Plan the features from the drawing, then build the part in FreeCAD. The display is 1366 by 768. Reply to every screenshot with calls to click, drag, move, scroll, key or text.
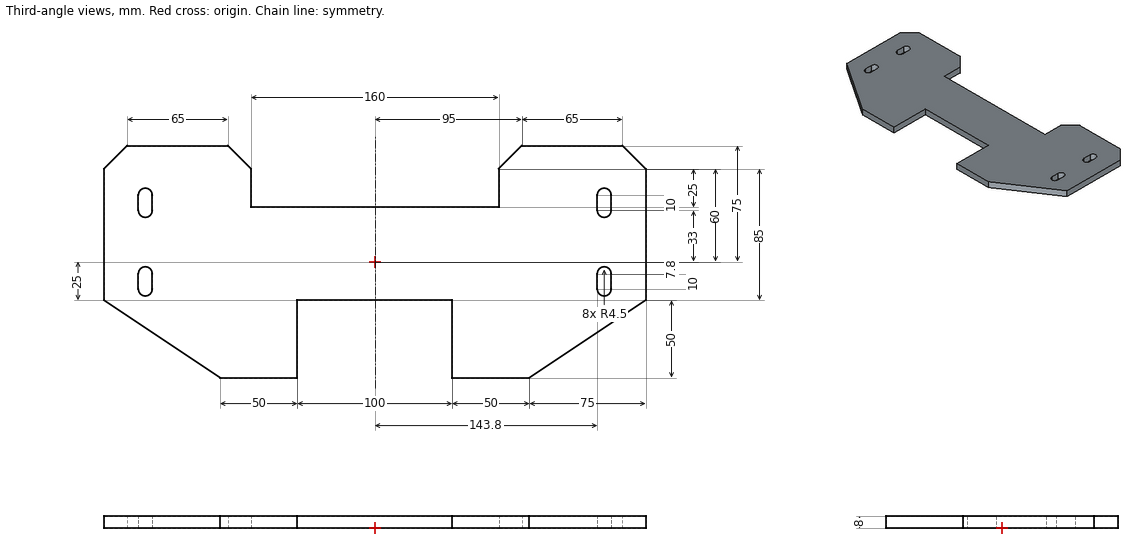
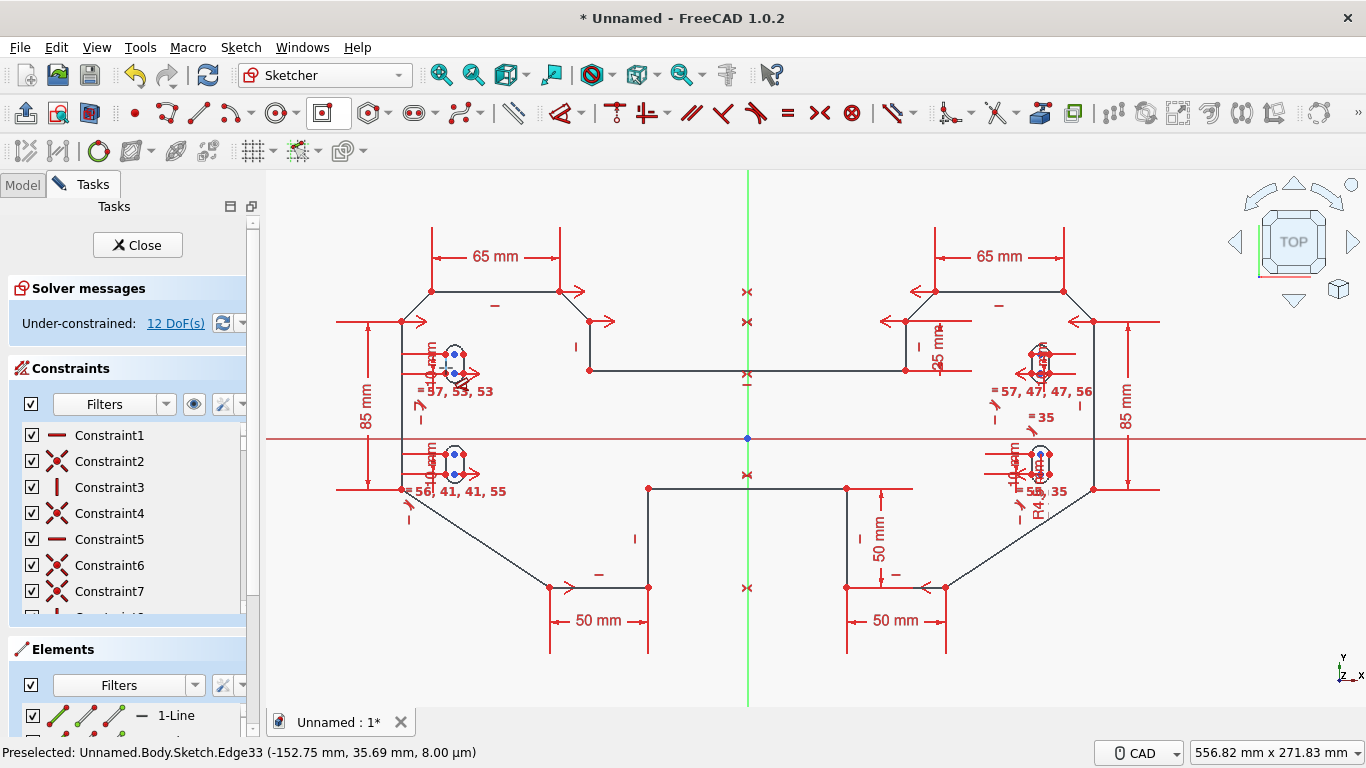
click(708, 489)
click(702, 523)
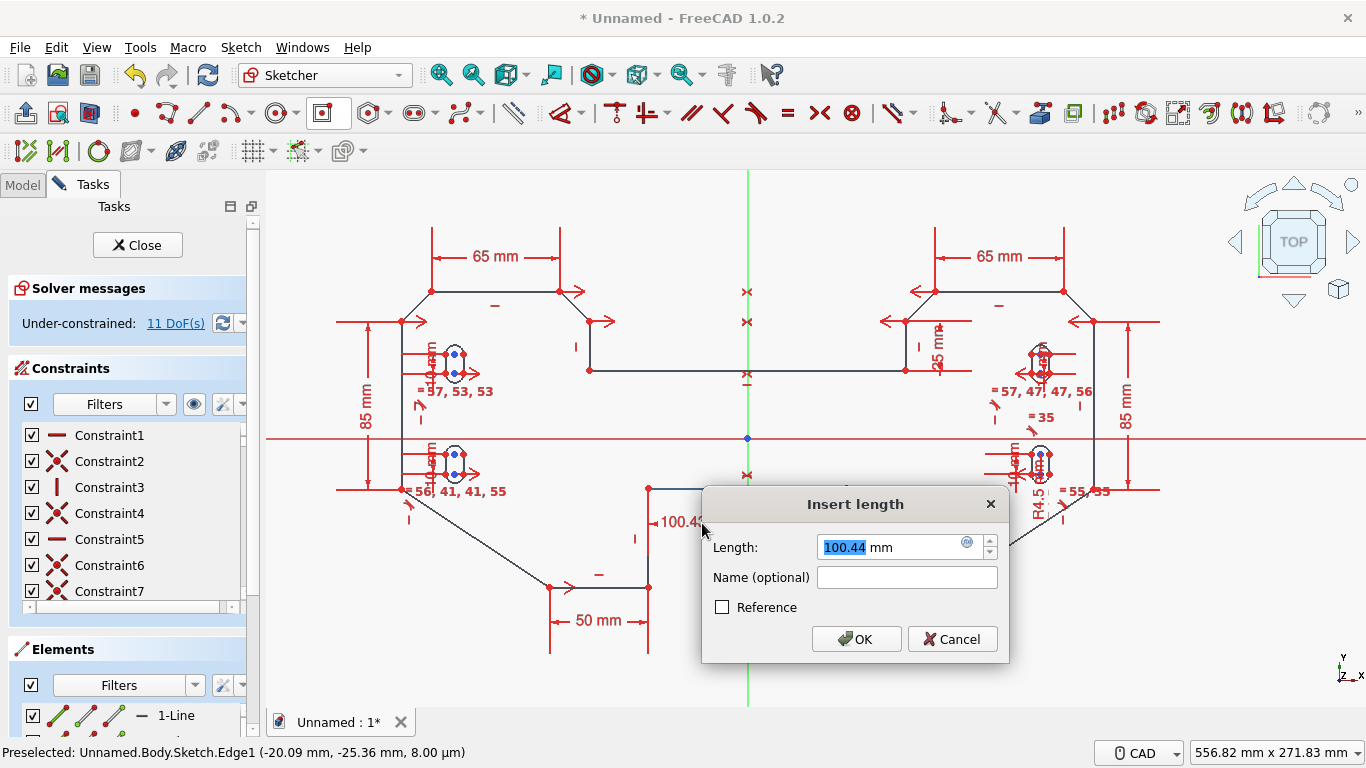
text(100)
key(Return)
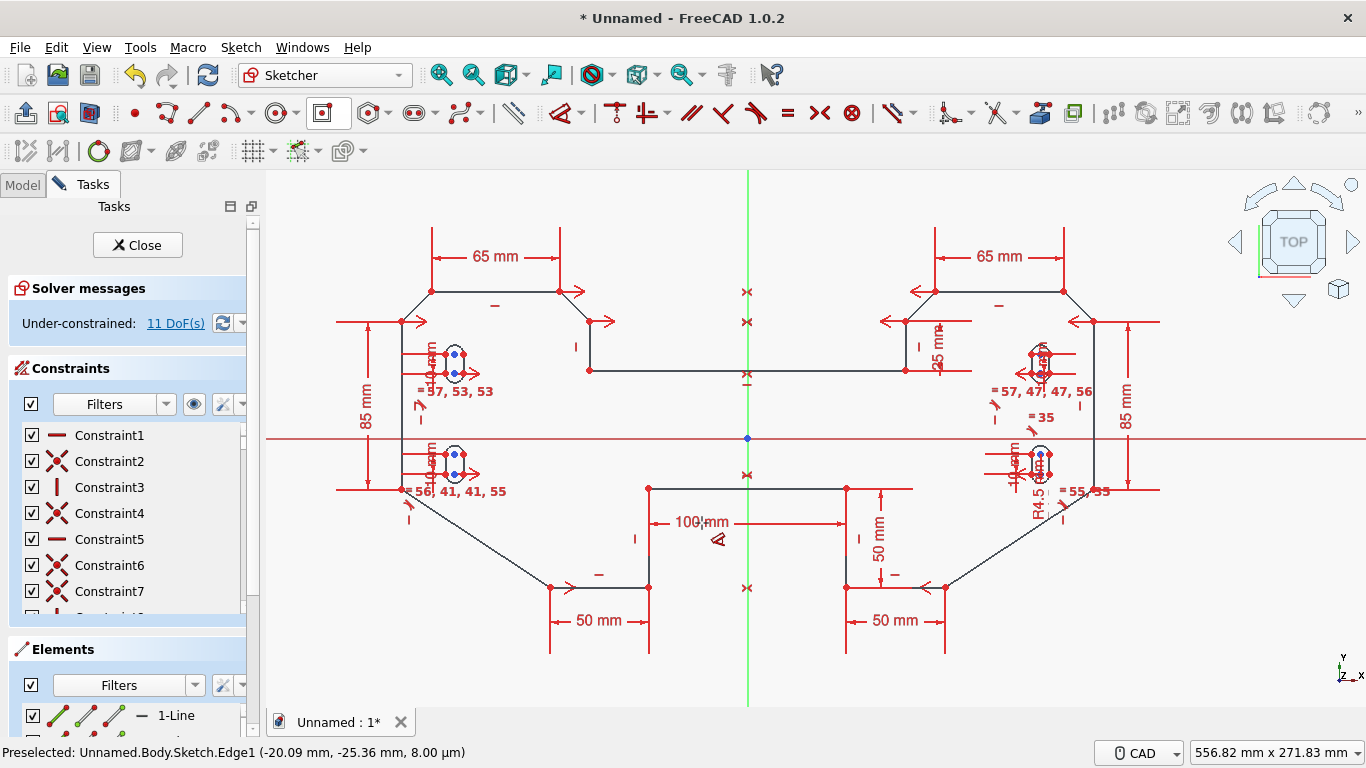
click(811, 371)
click(675, 337)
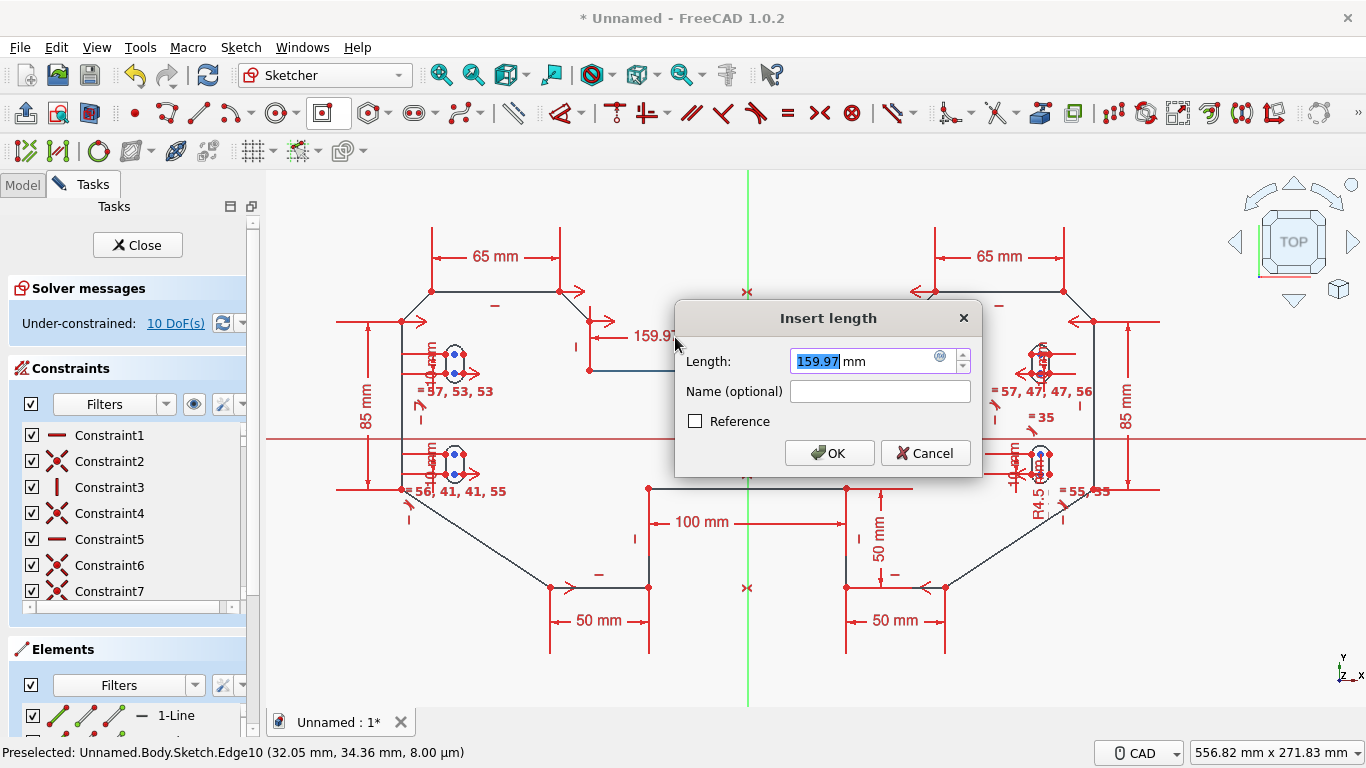
text(160)
key(Return)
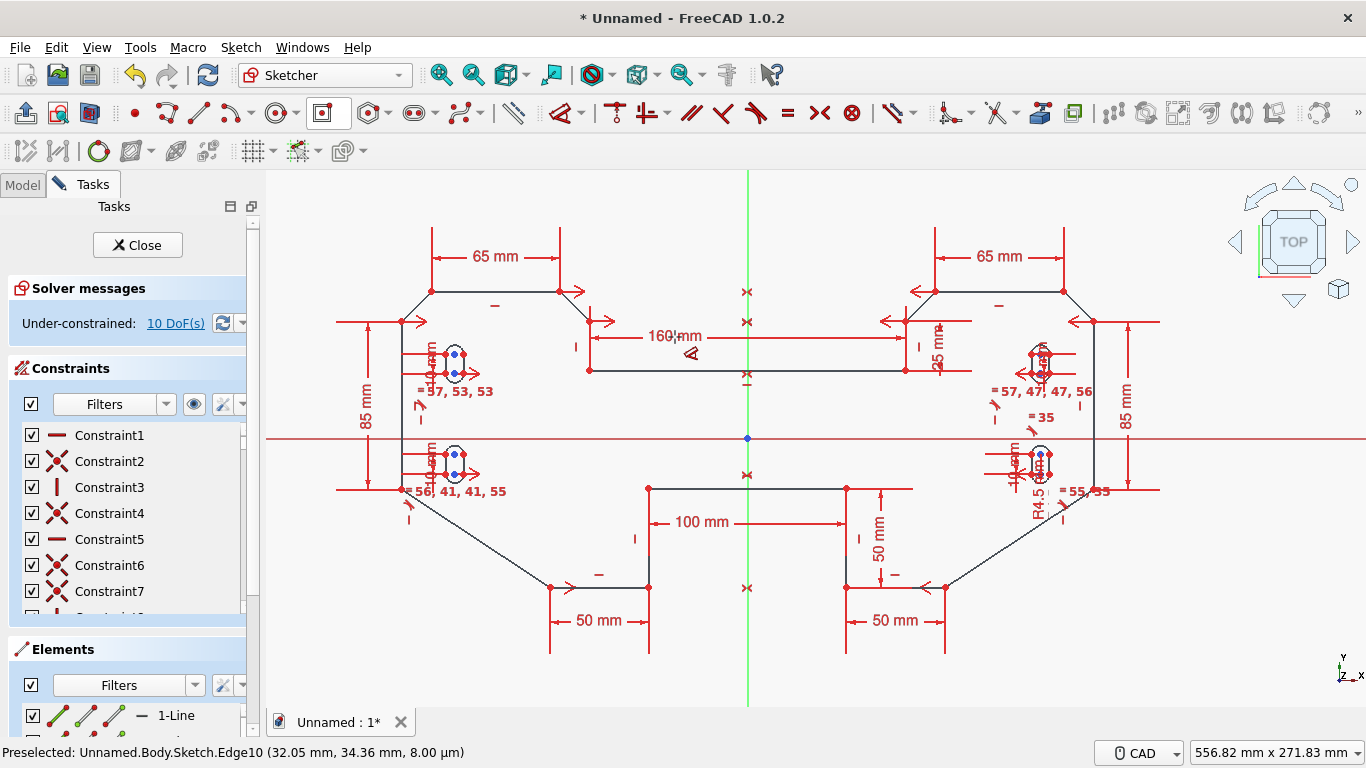
click(649, 489)
click(615, 464)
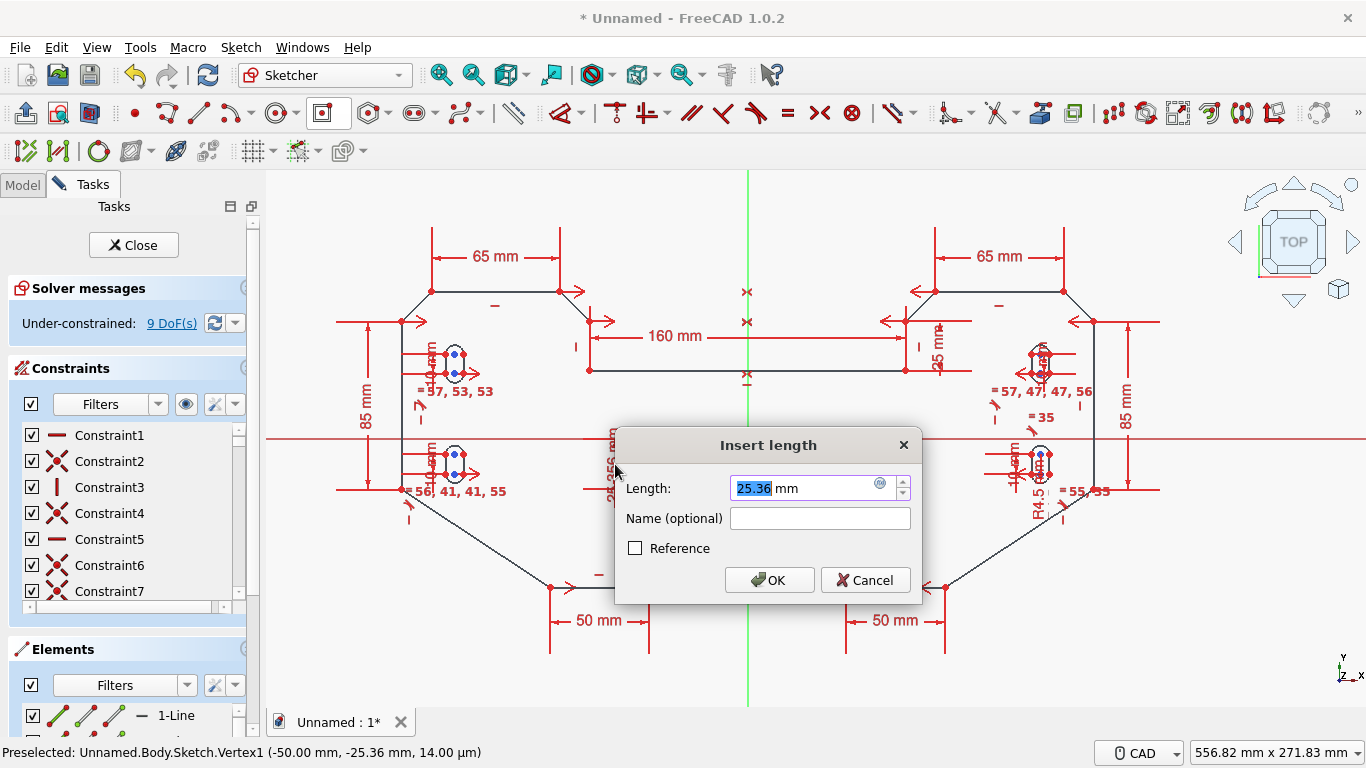
text(25)
key(Return)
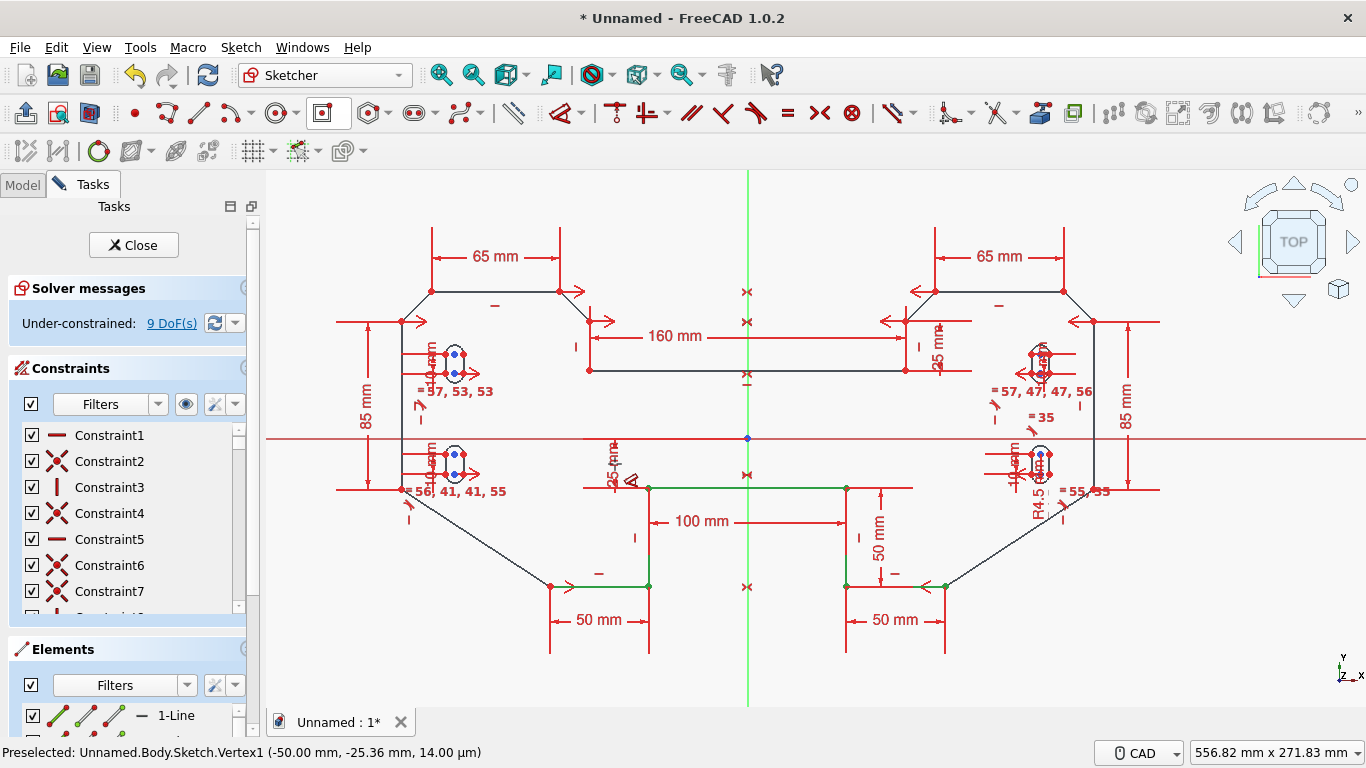
click(1094, 490)
click(1128, 464)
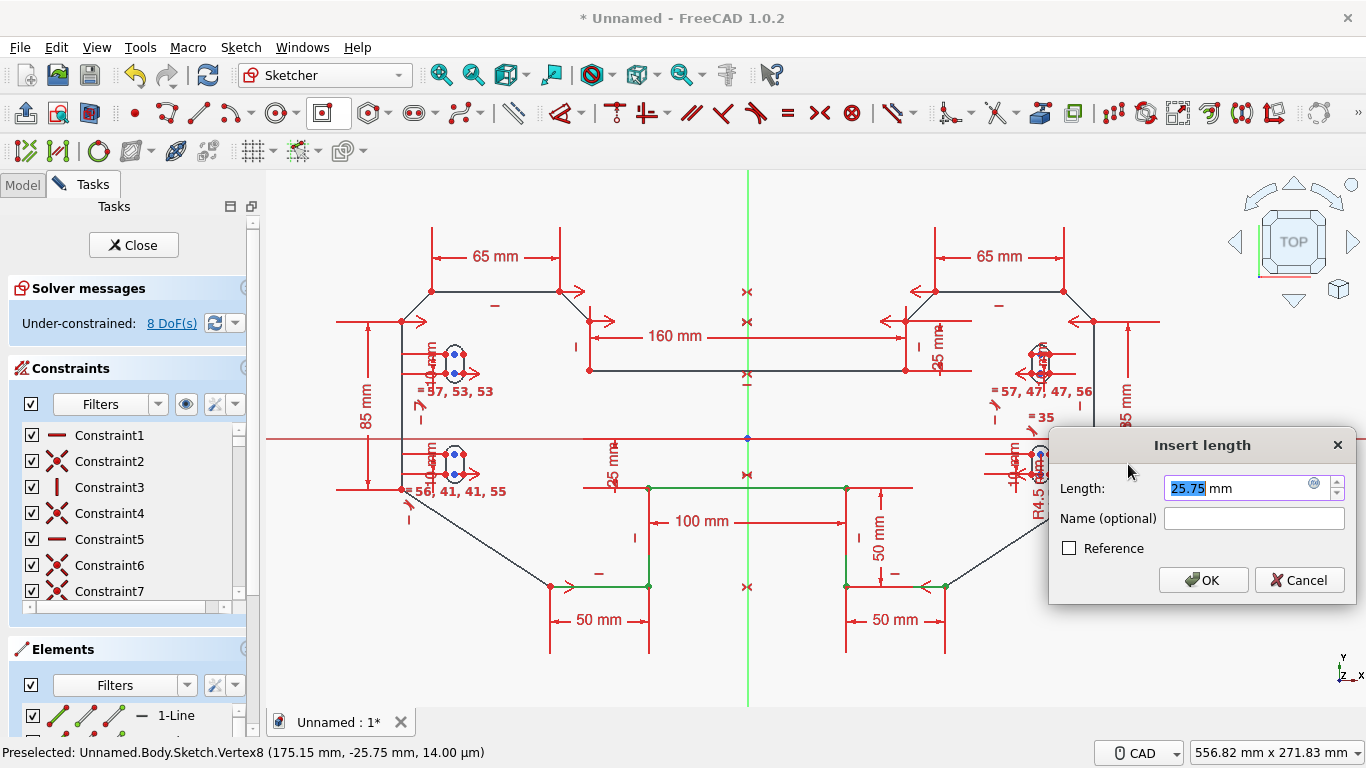
text(25)
key(Return)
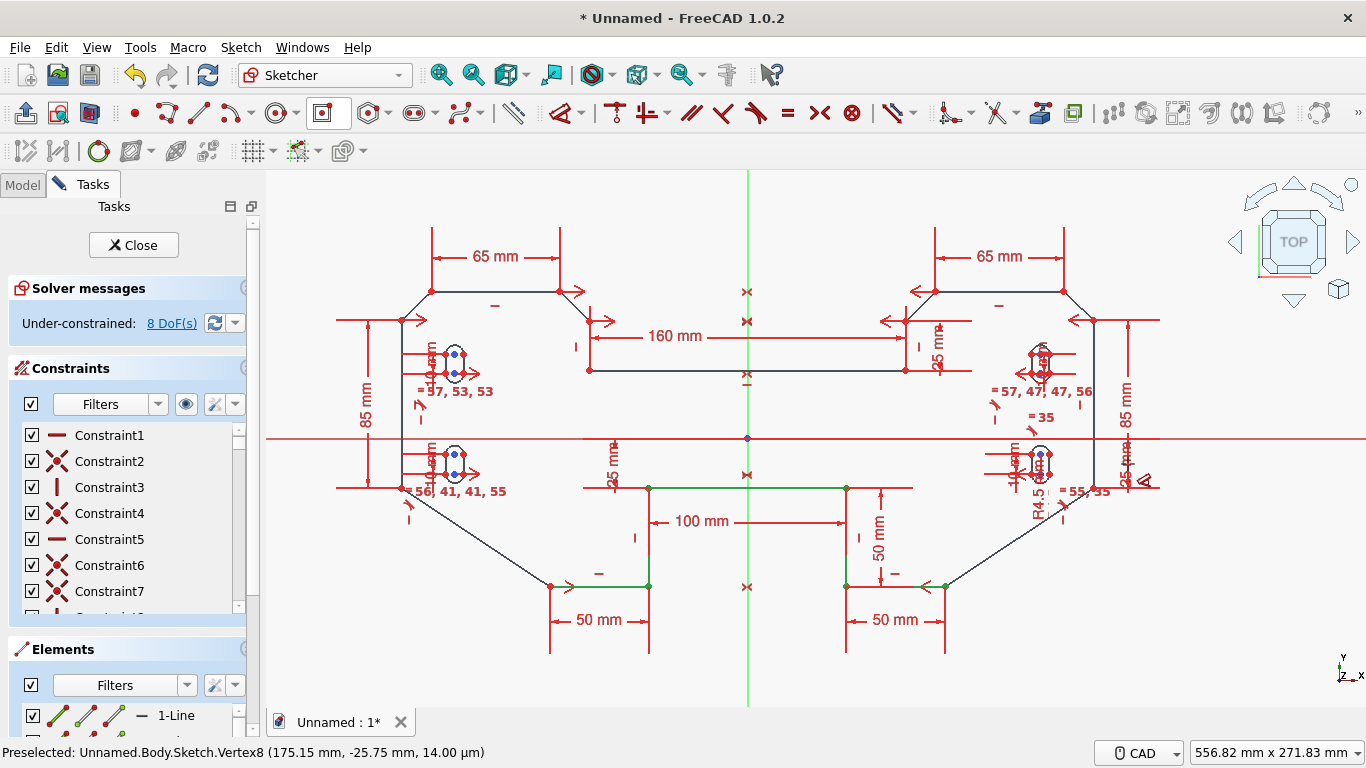
click(1064, 292)
click(714, 399)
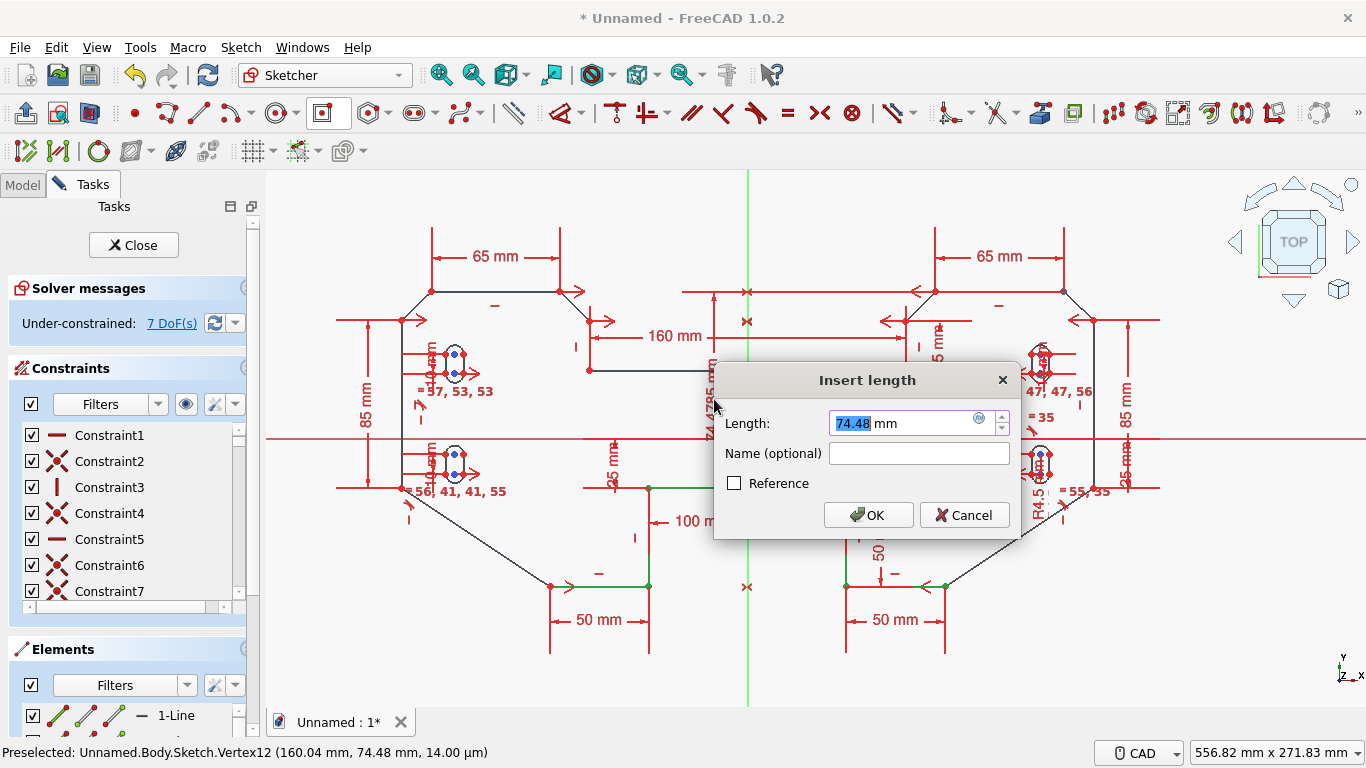
text(75)
key(Return)